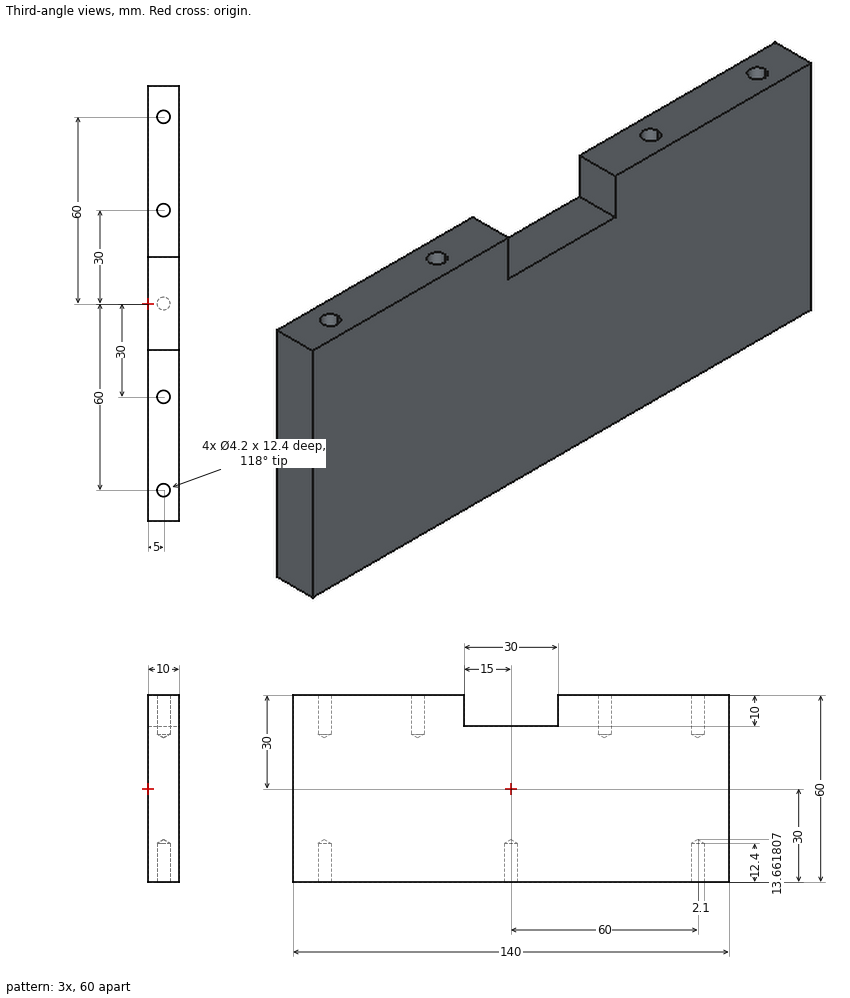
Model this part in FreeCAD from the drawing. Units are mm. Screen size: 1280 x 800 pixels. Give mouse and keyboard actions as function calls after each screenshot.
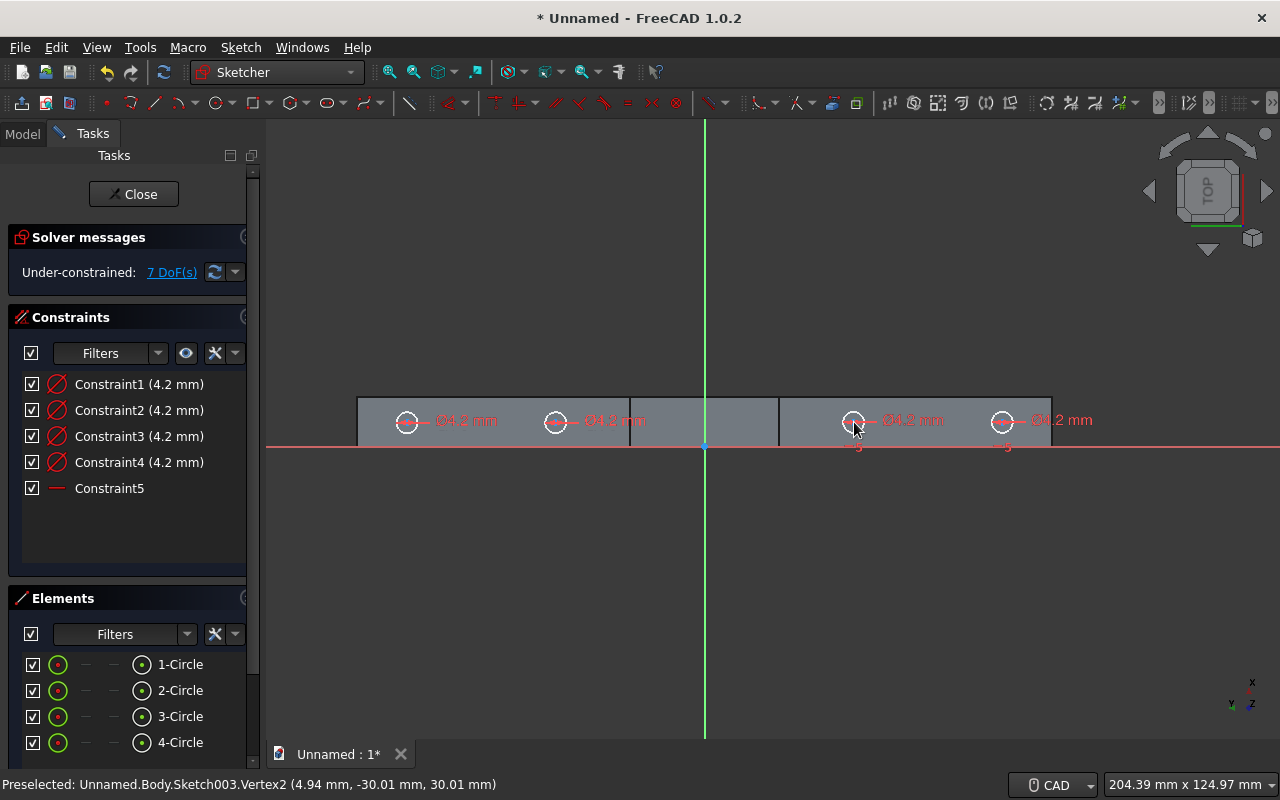
click(854, 422)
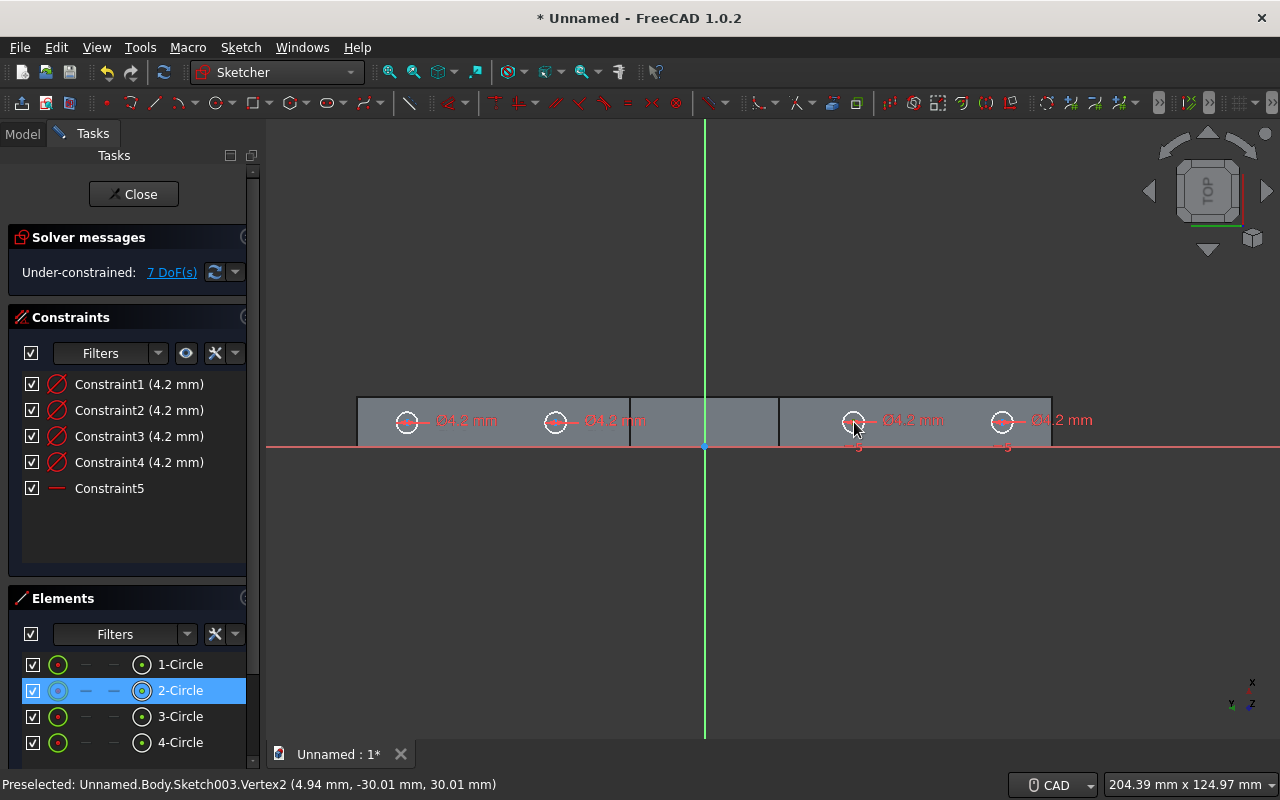
click(556, 423)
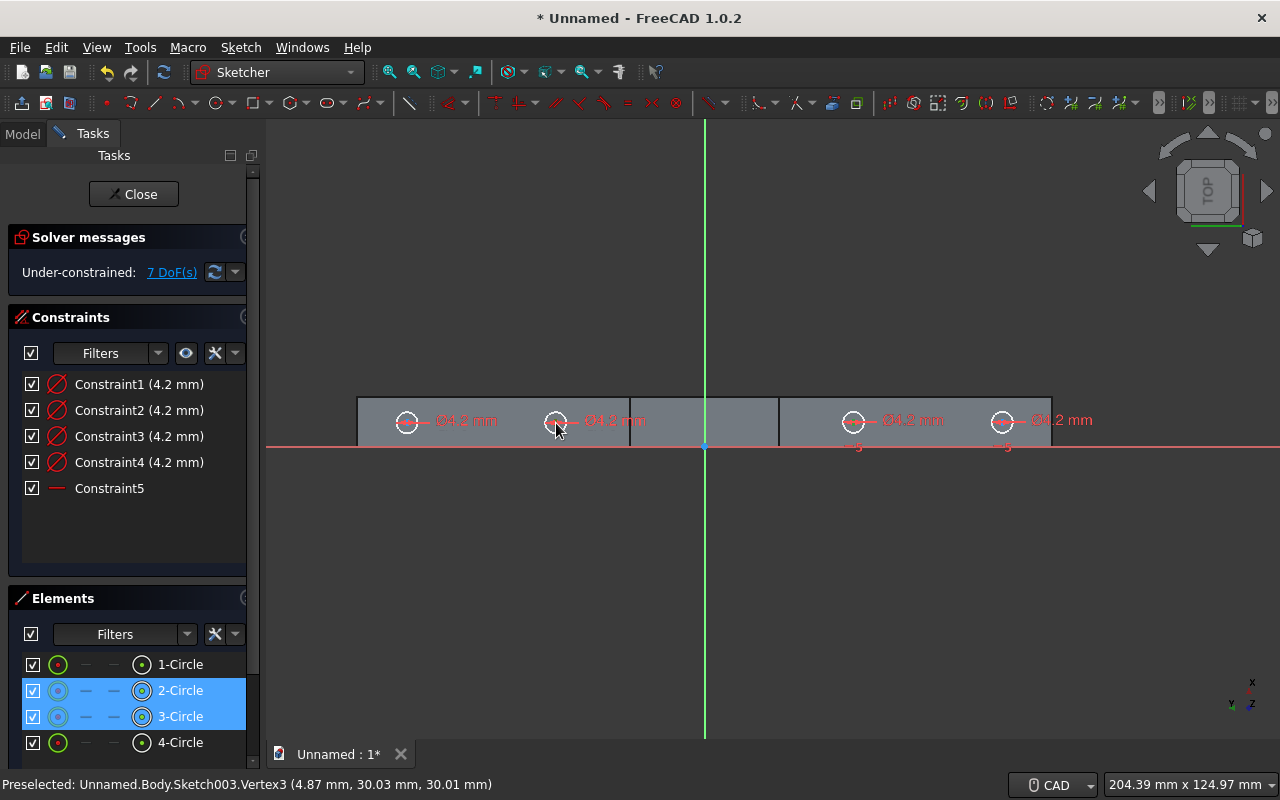
key(h)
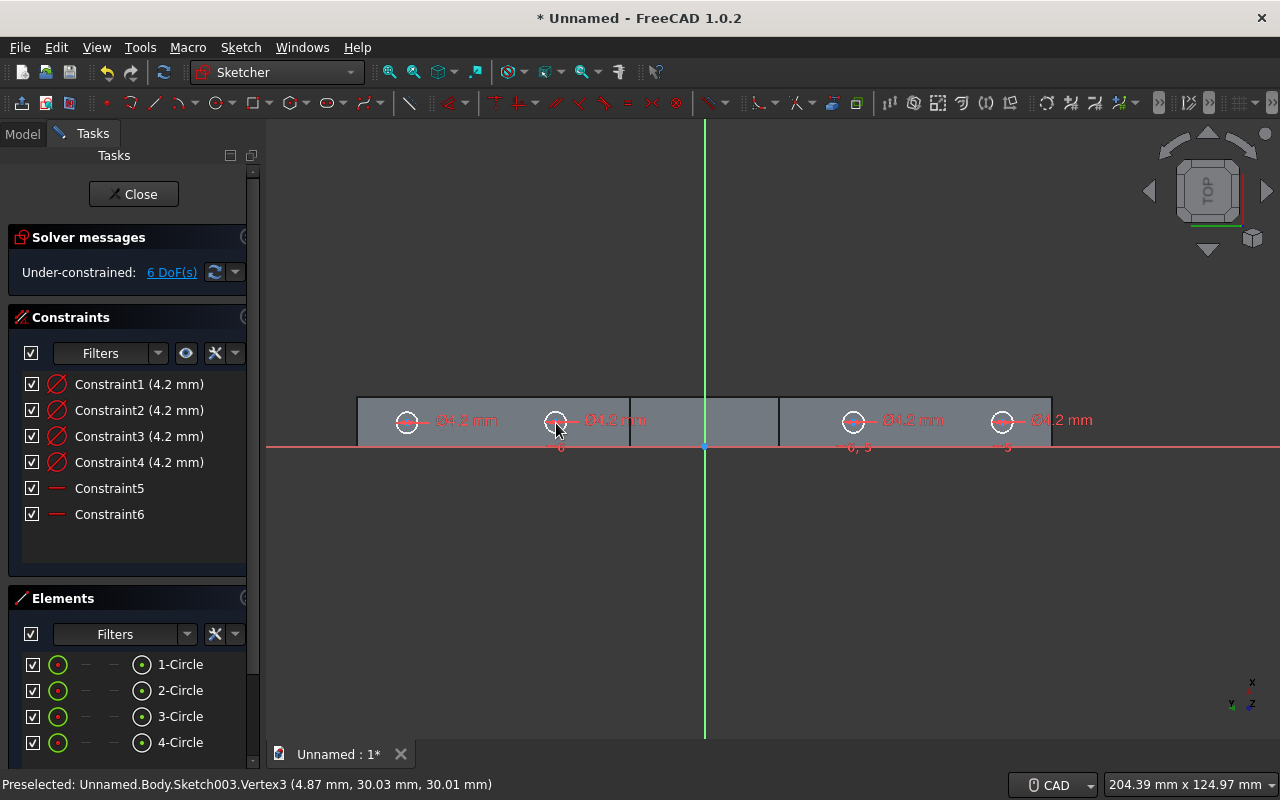
click(556, 422)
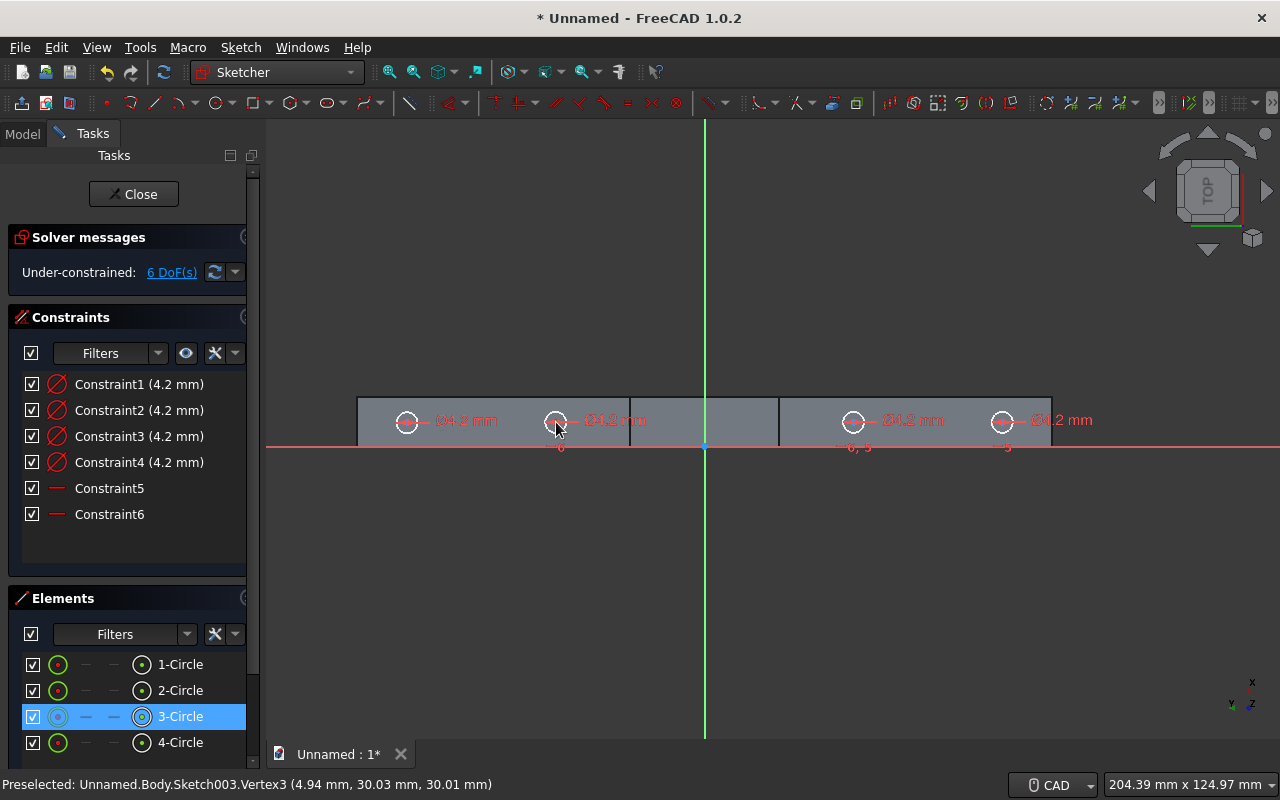
click(407, 423)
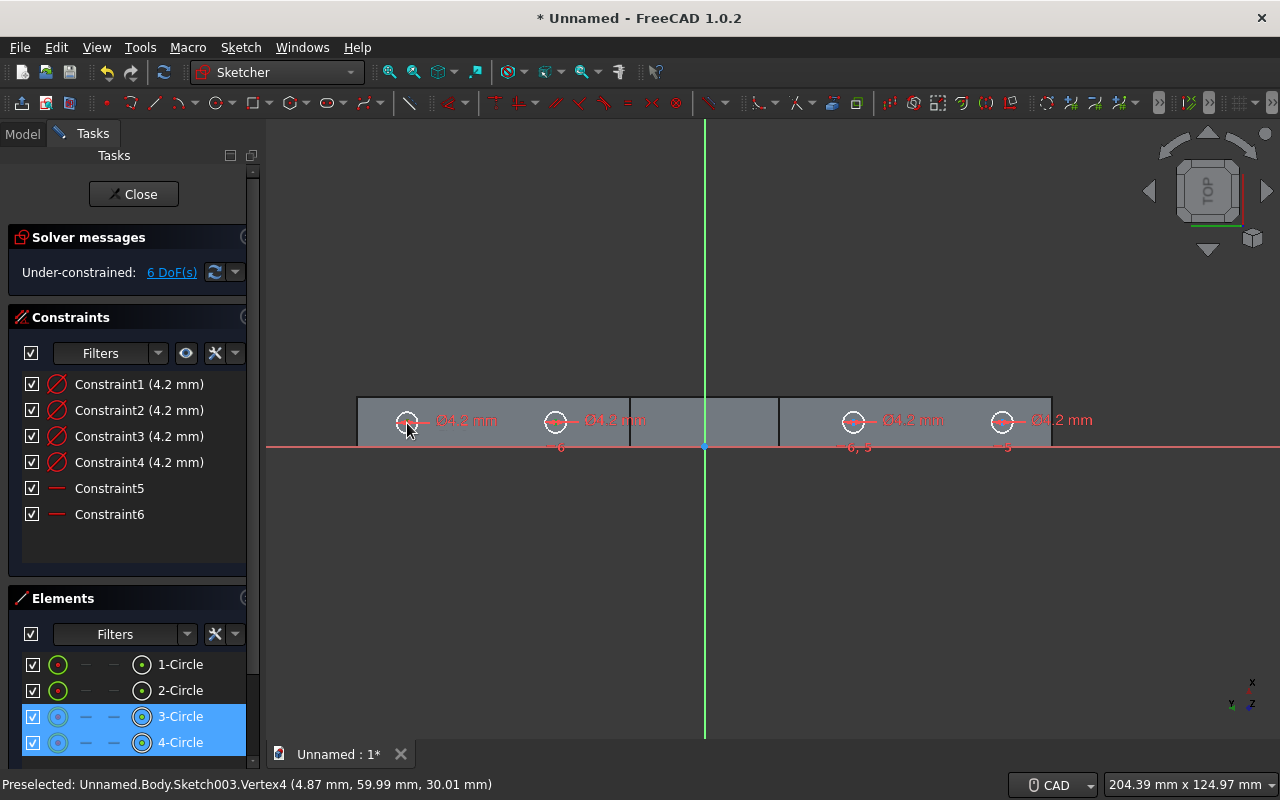
click(538, 104)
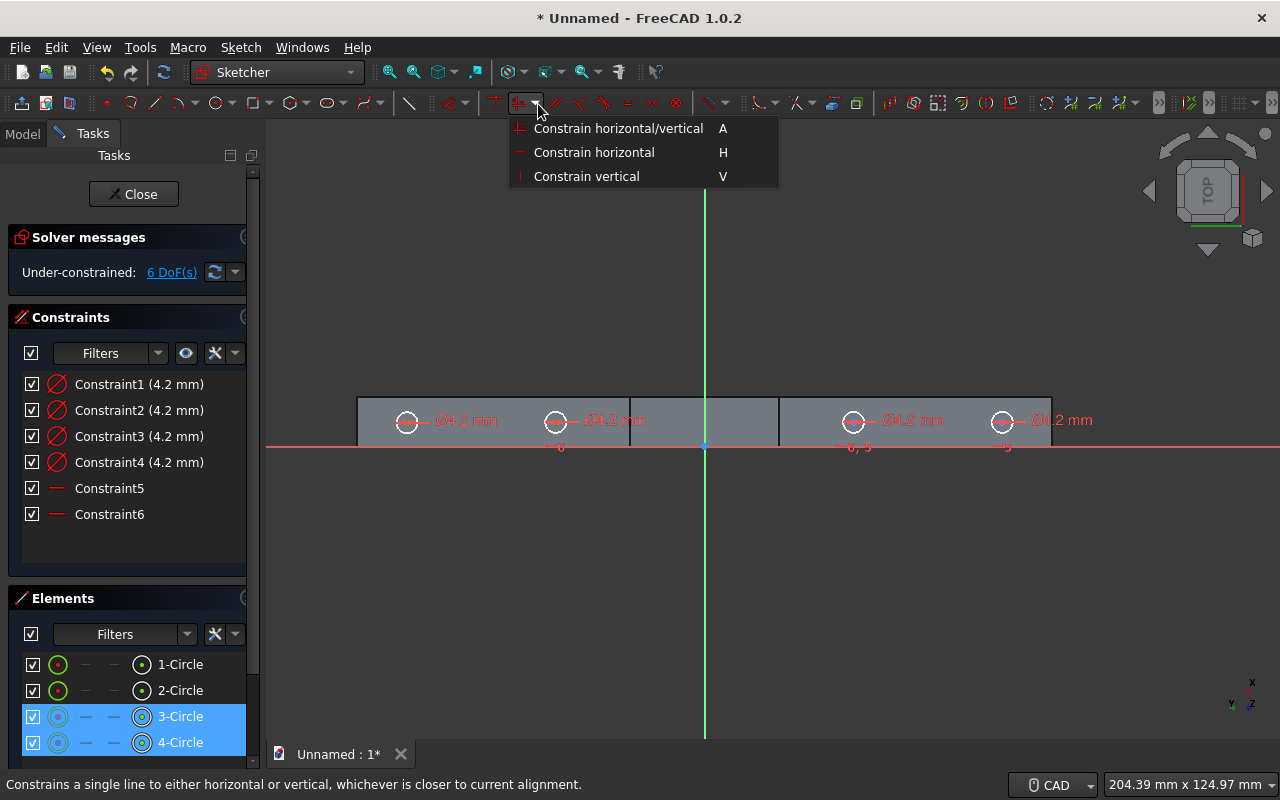
click(644, 152)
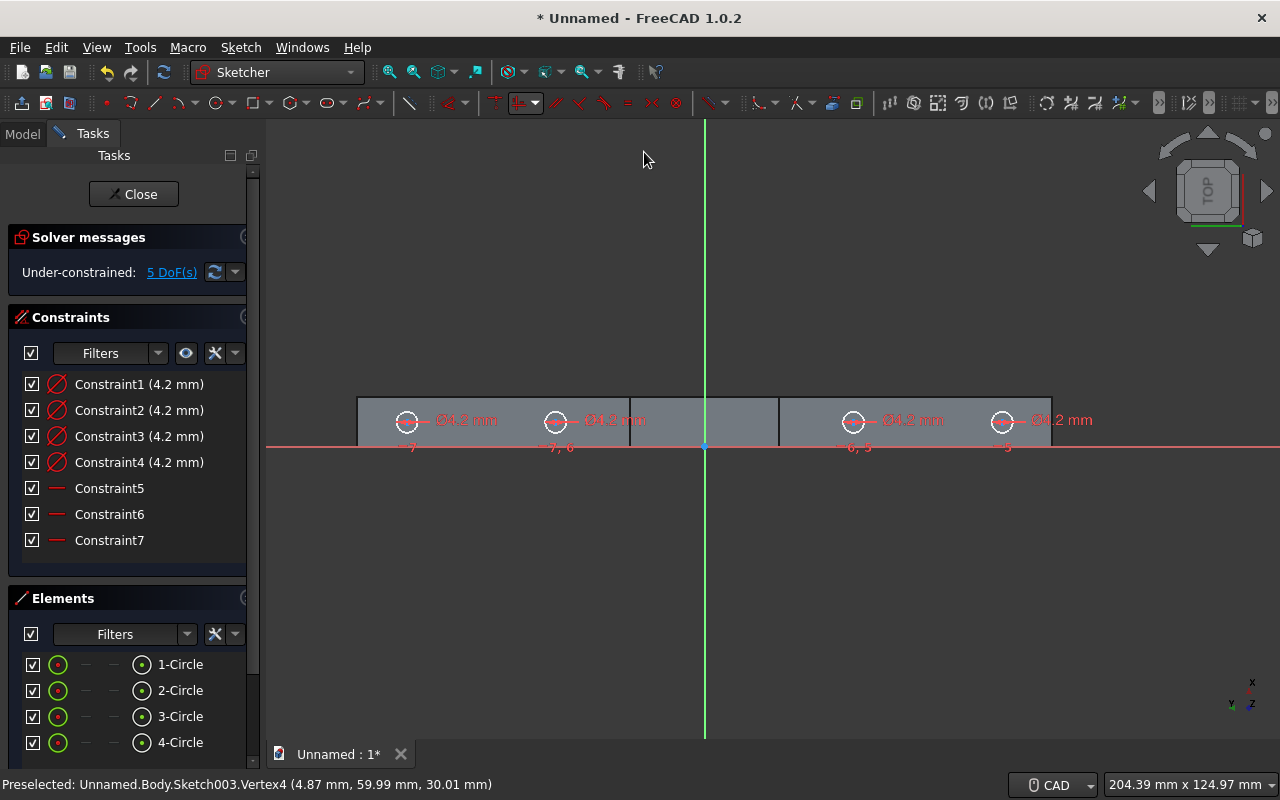
click(448, 104)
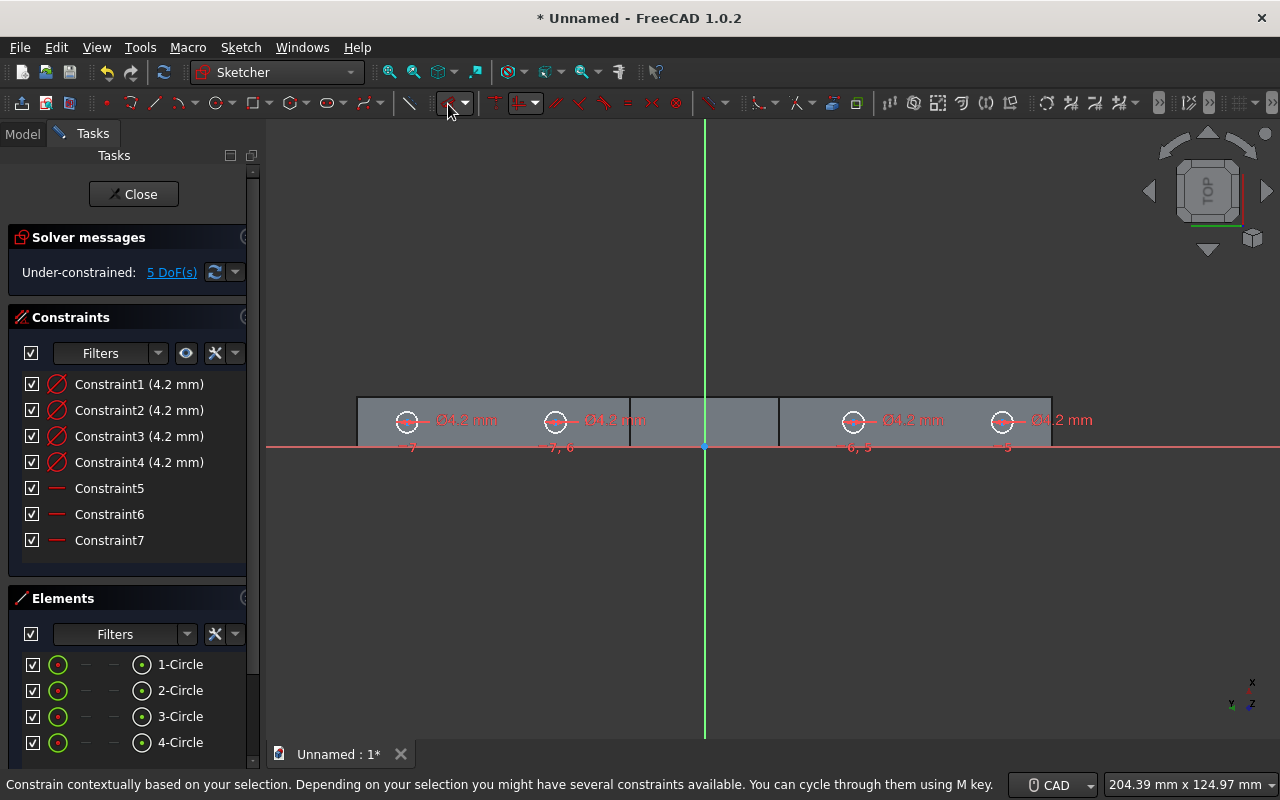
scroll(1002, 422, up, 3)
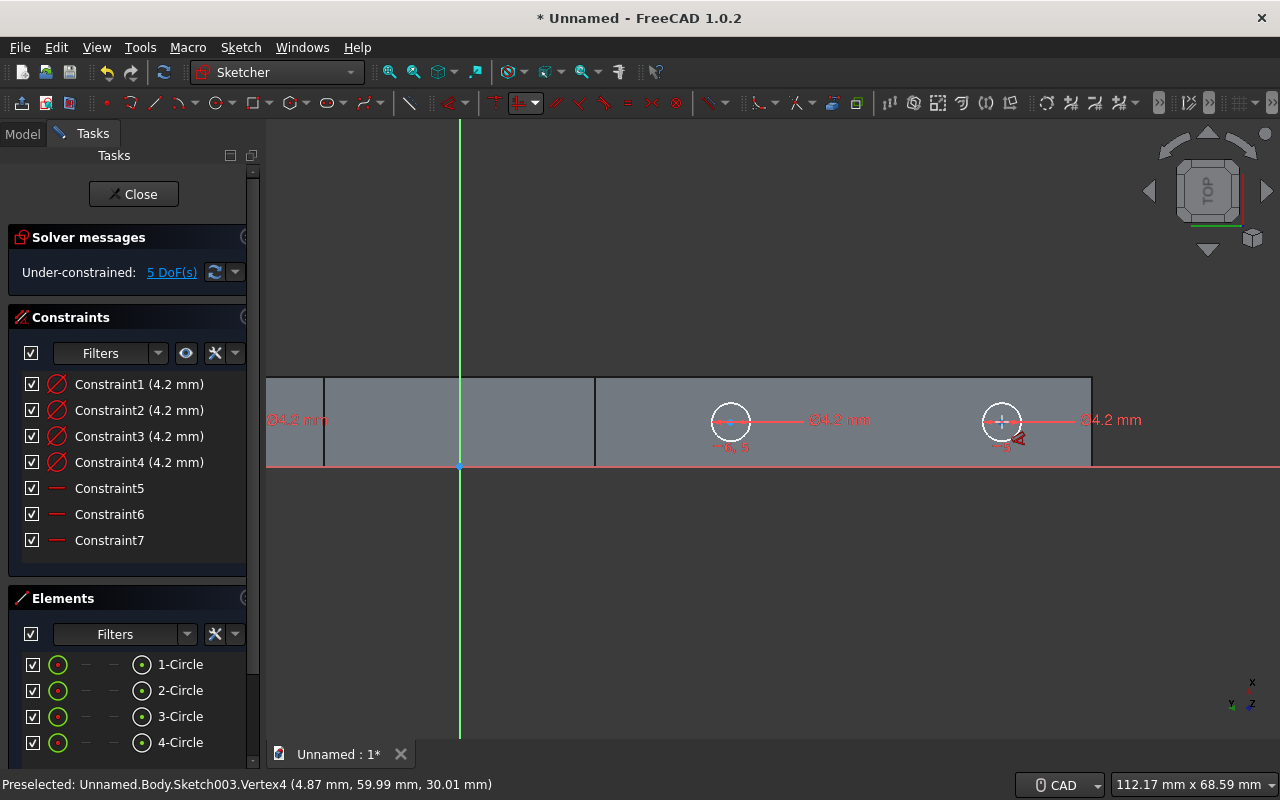
click(1002, 422)
click(1036, 445)